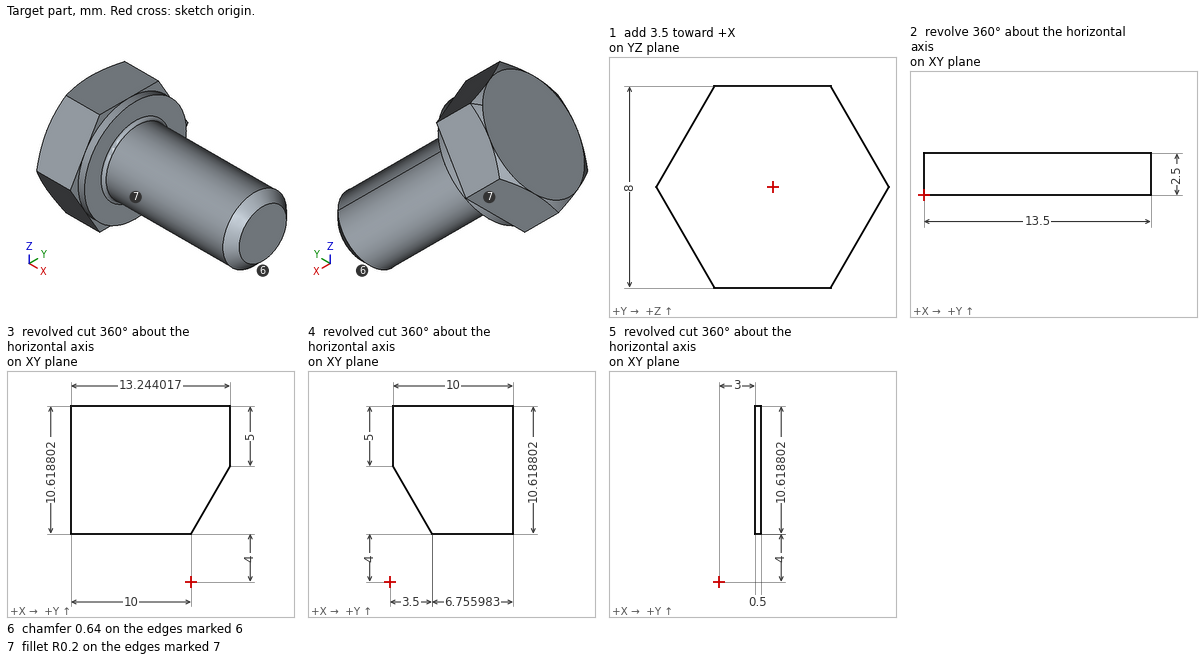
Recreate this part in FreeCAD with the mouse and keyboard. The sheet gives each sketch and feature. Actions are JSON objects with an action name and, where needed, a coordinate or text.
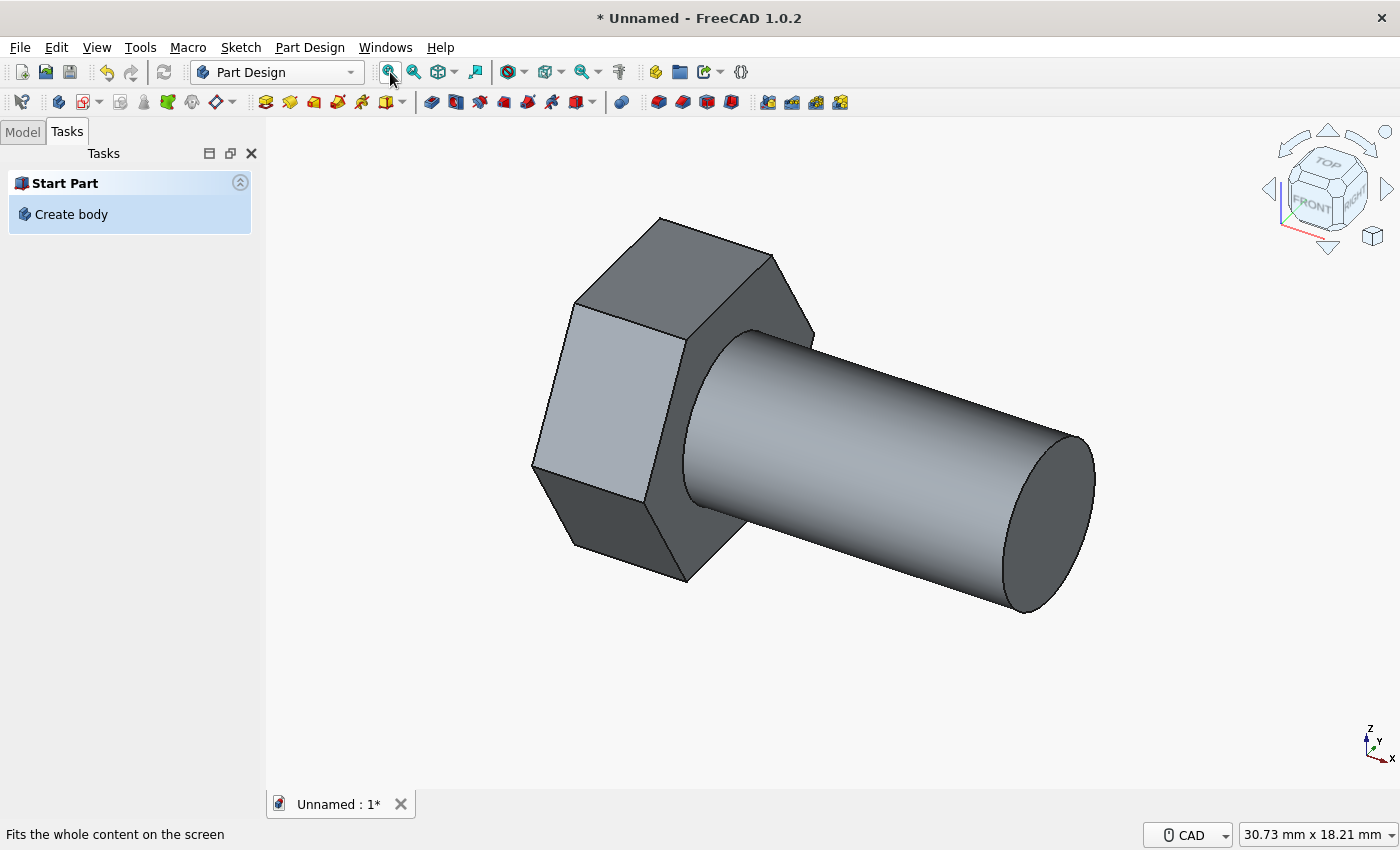
{"action": "left_click", "coordinate": [84, 102]}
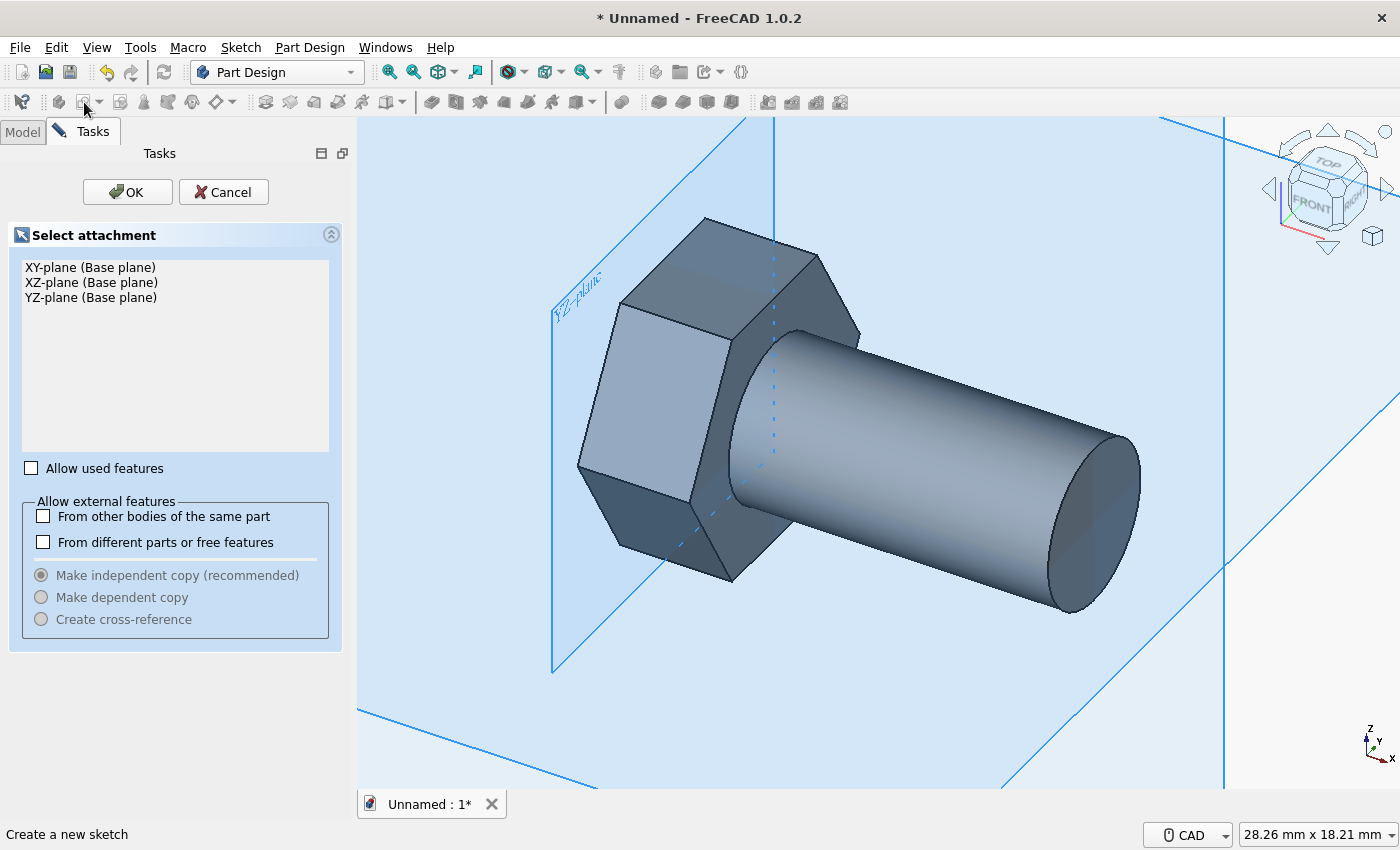
{"action": "left_click", "coordinate": [82, 268]}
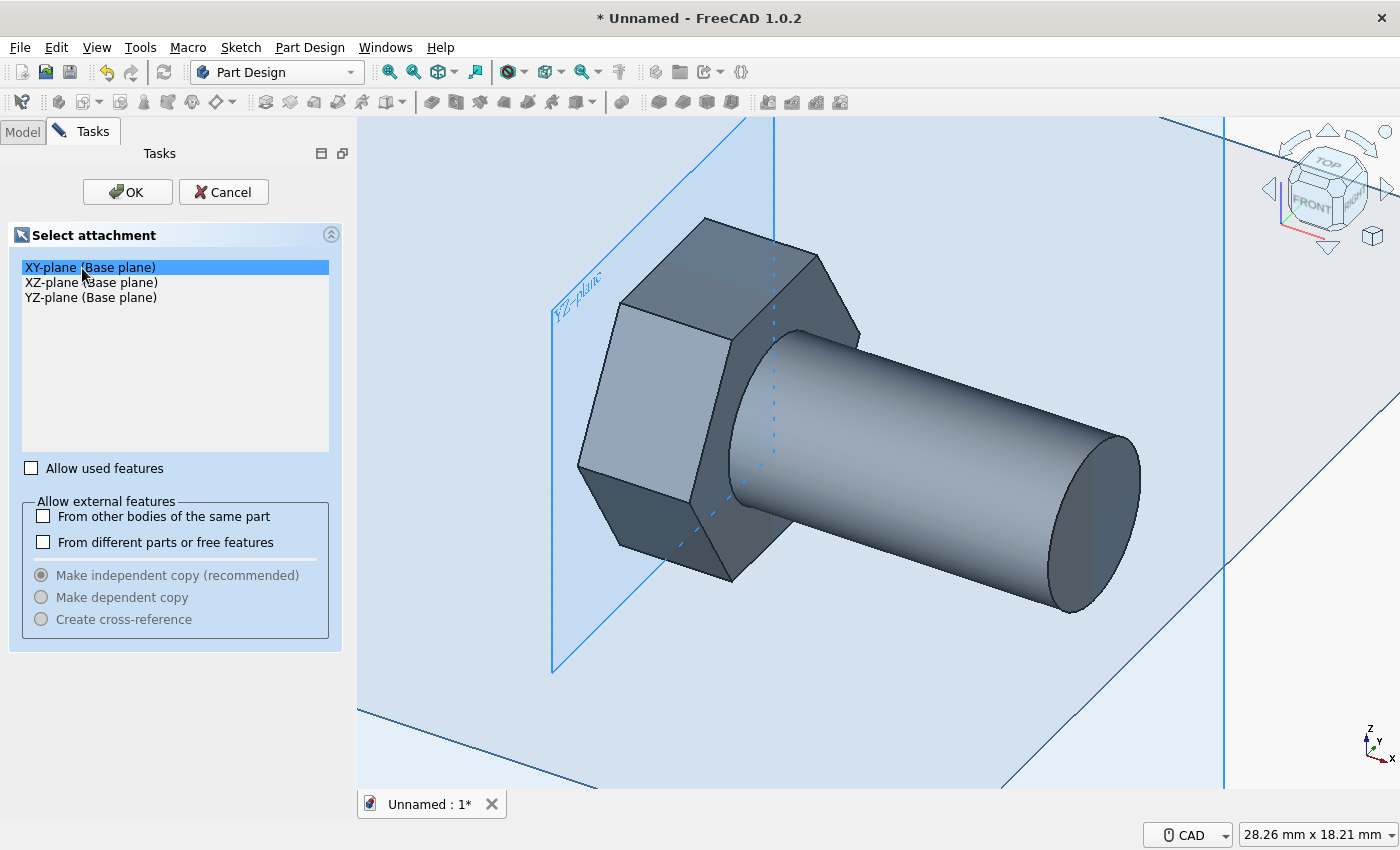
{"action": "left_click", "coordinate": [128, 192]}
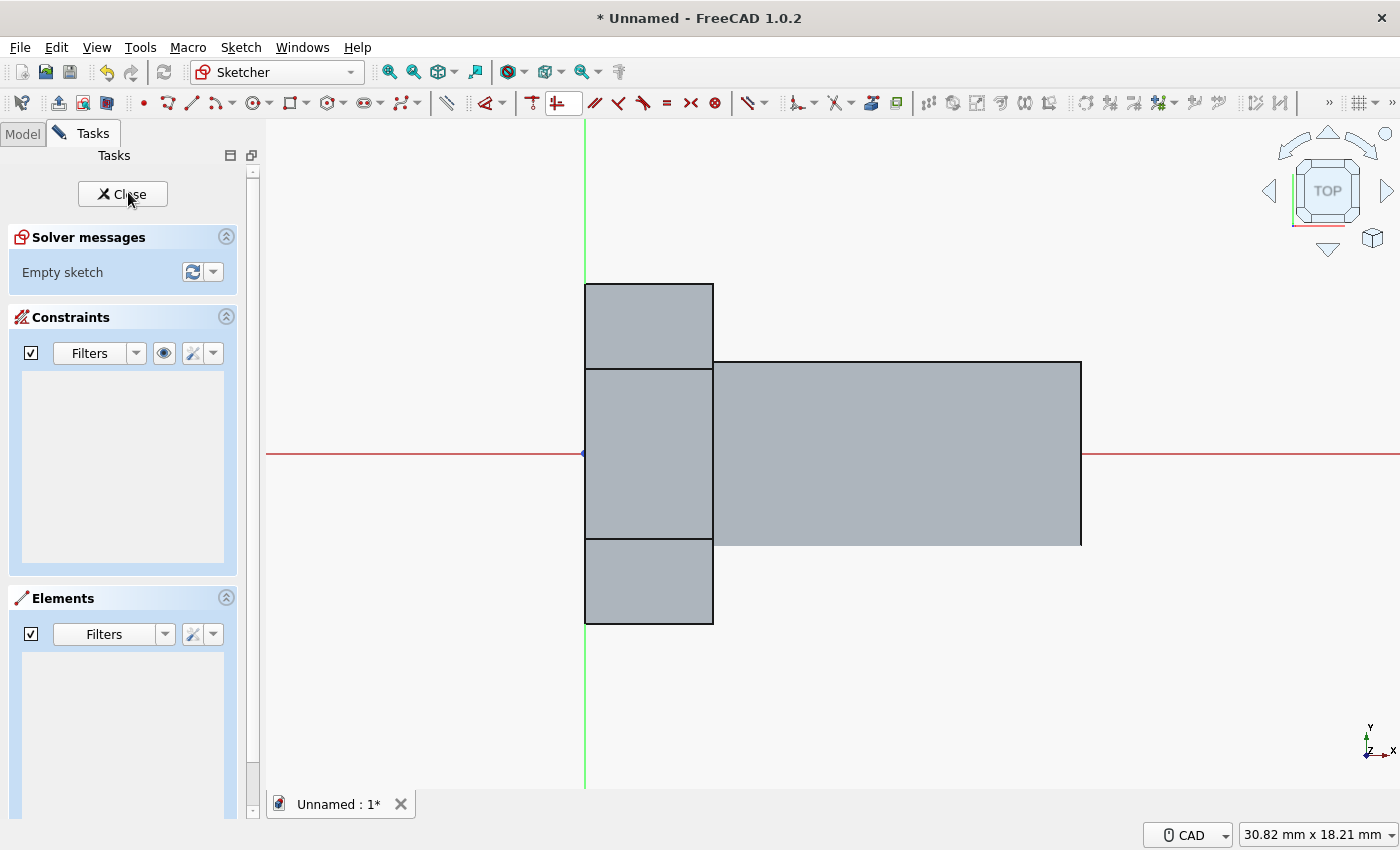
{"action": "left_click", "coordinate": [108, 104]}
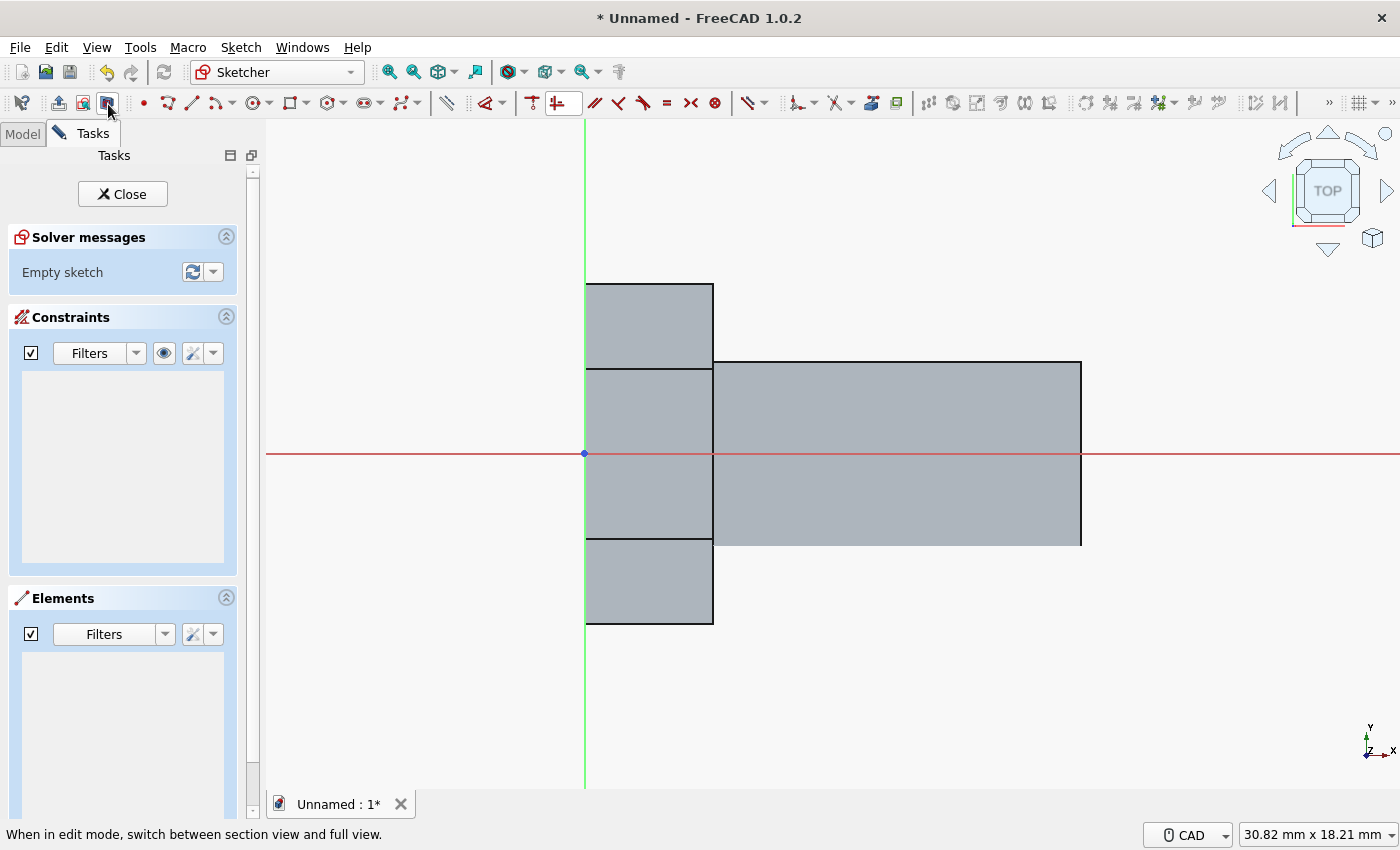
{"action": "scroll", "coordinate": [1235, 761], "scroll_direction": "down", "scroll_amount": 2}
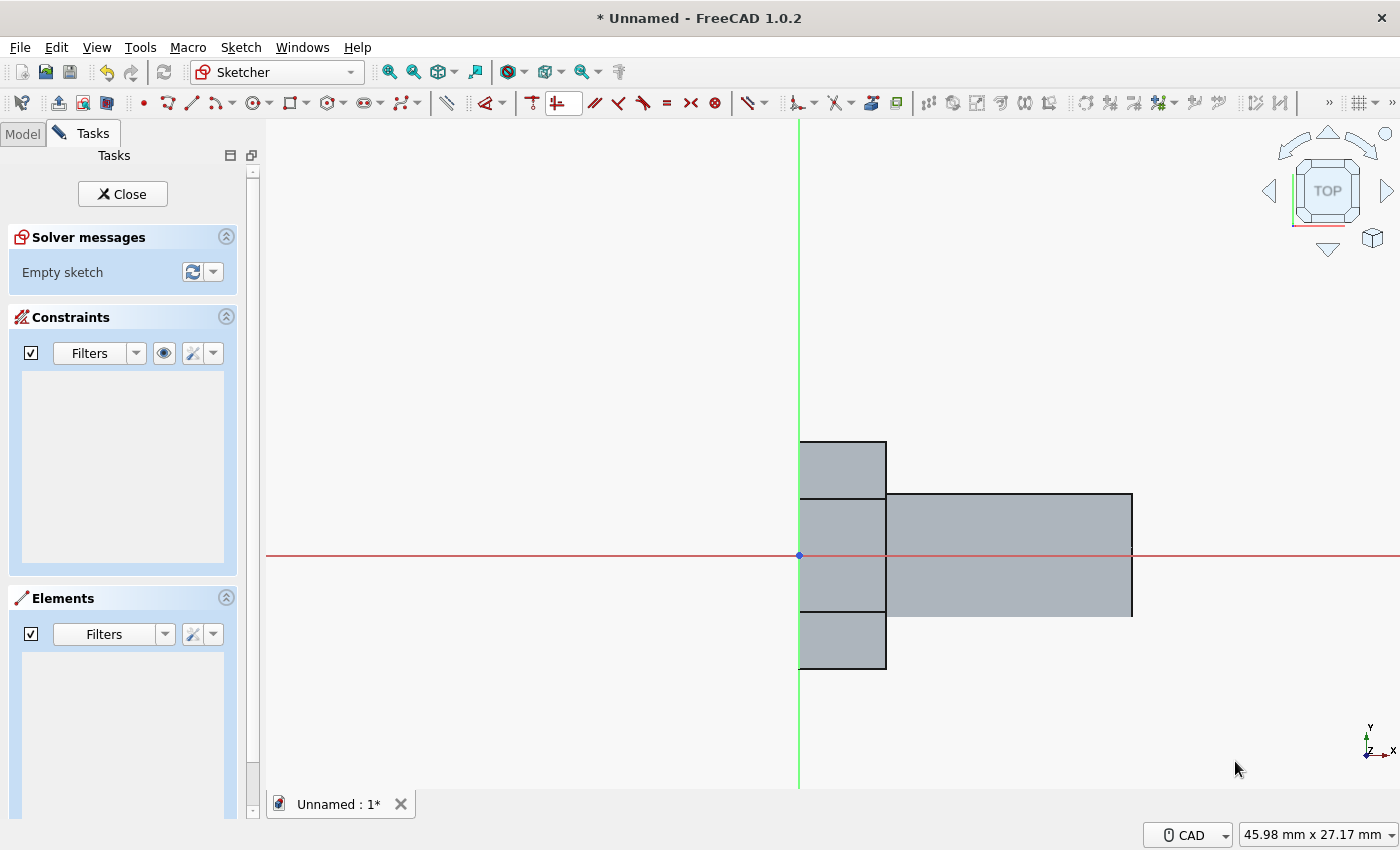
{"action": "left_click", "coordinate": [168, 104]}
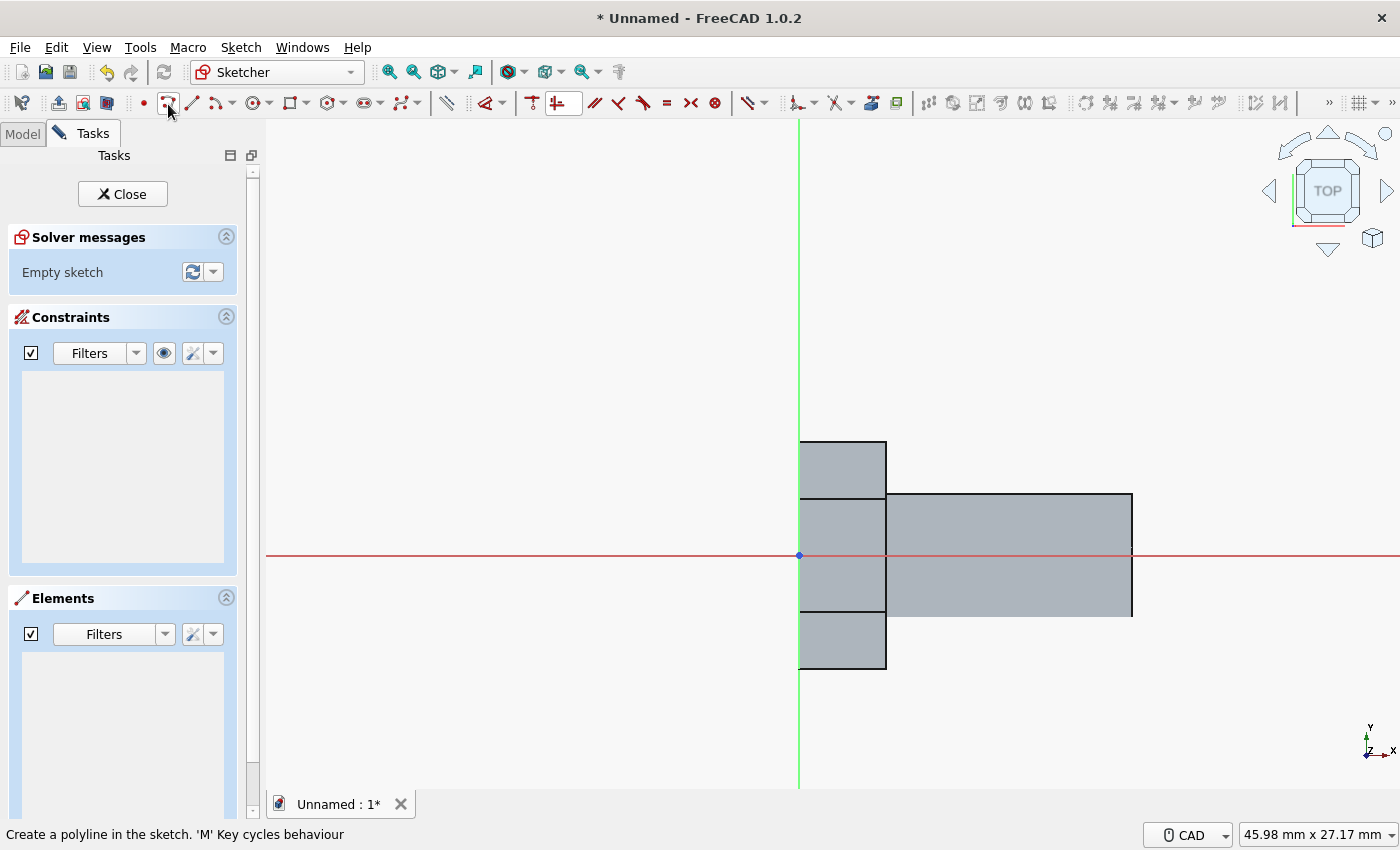
{"action": "left_click", "coordinate": [799, 457]}
{"action": "left_click", "coordinate": [879, 318]}
{"action": "left_click", "coordinate": [879, 195]}
{"action": "left_click", "coordinate": [553, 195]}
{"action": "left_click", "coordinate": [553, 457]}
{"action": "left_click", "coordinate": [799, 458]}
{"action": "key", "text": "Escape"}
{"action": "key", "text": "Escape"}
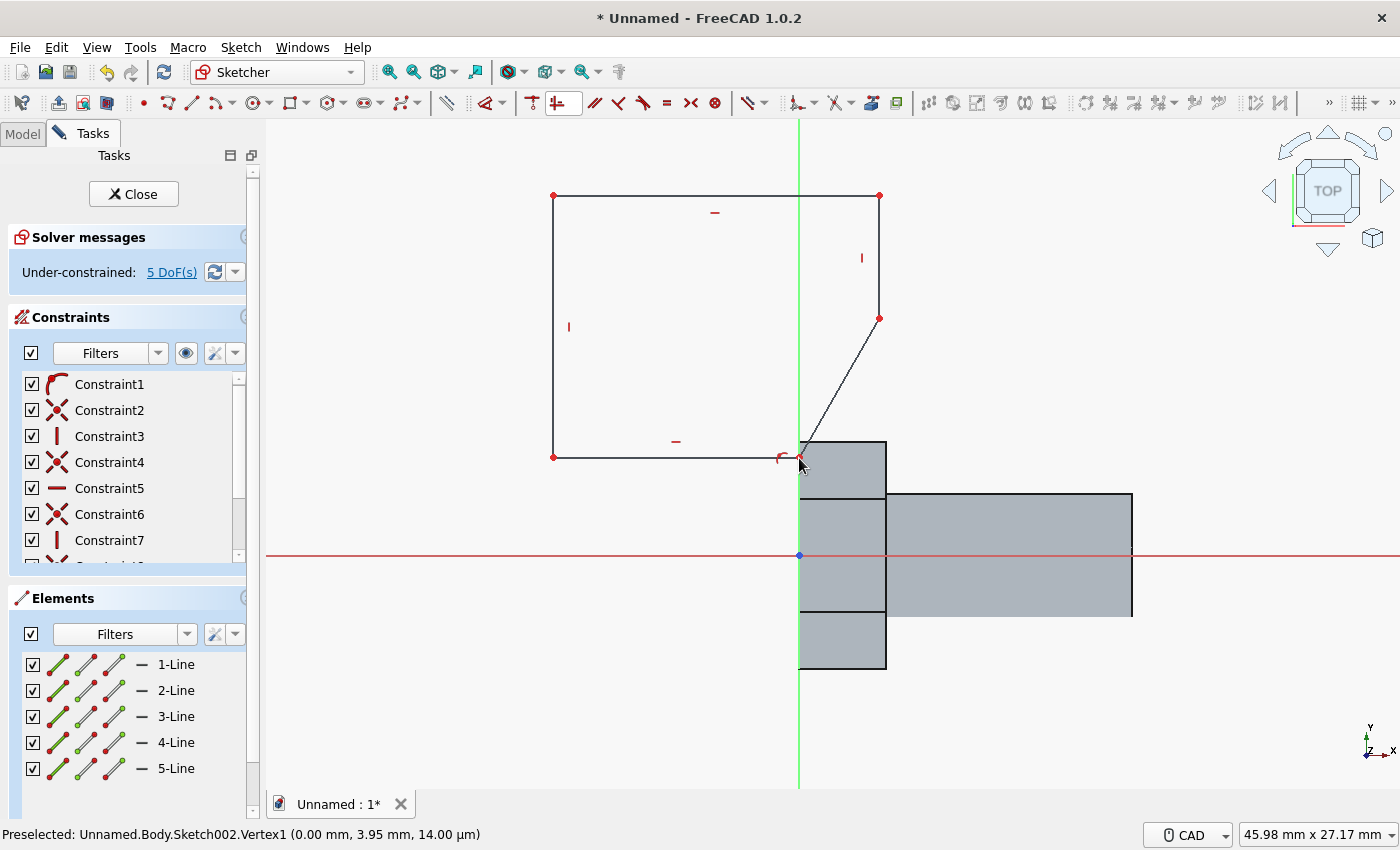
{"action": "left_click", "coordinate": [879, 282]}